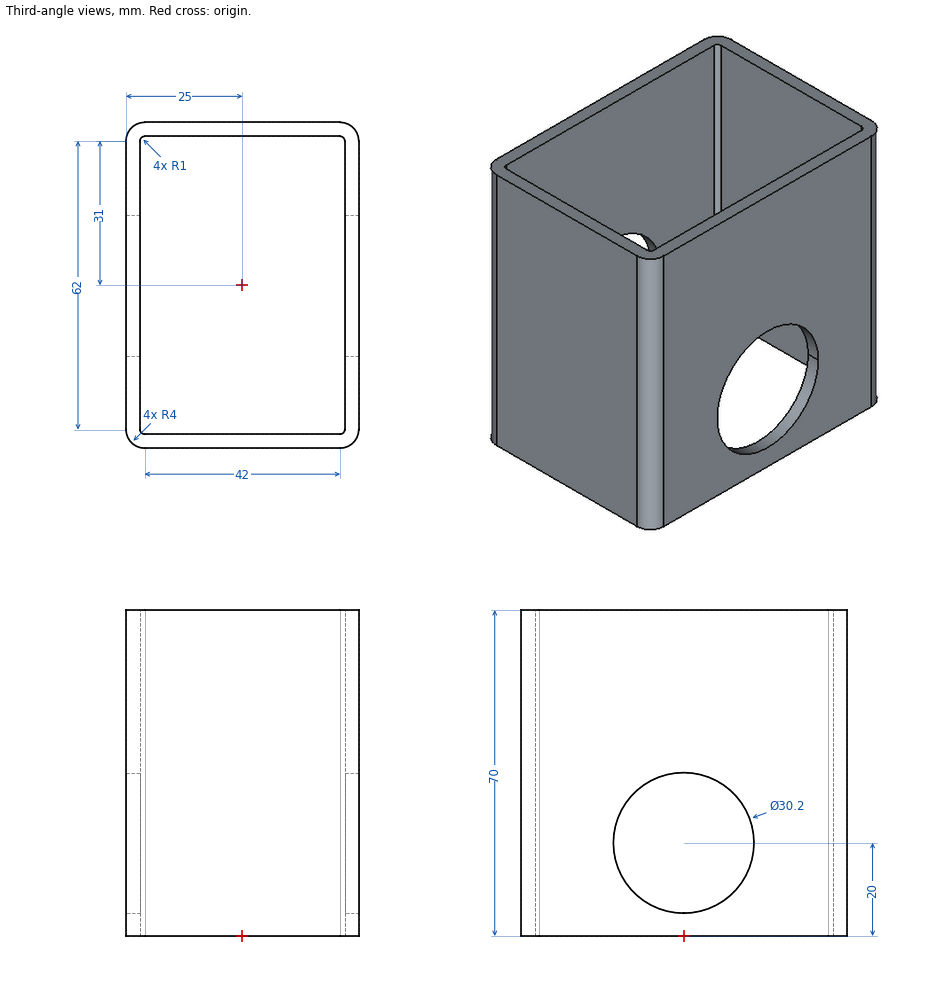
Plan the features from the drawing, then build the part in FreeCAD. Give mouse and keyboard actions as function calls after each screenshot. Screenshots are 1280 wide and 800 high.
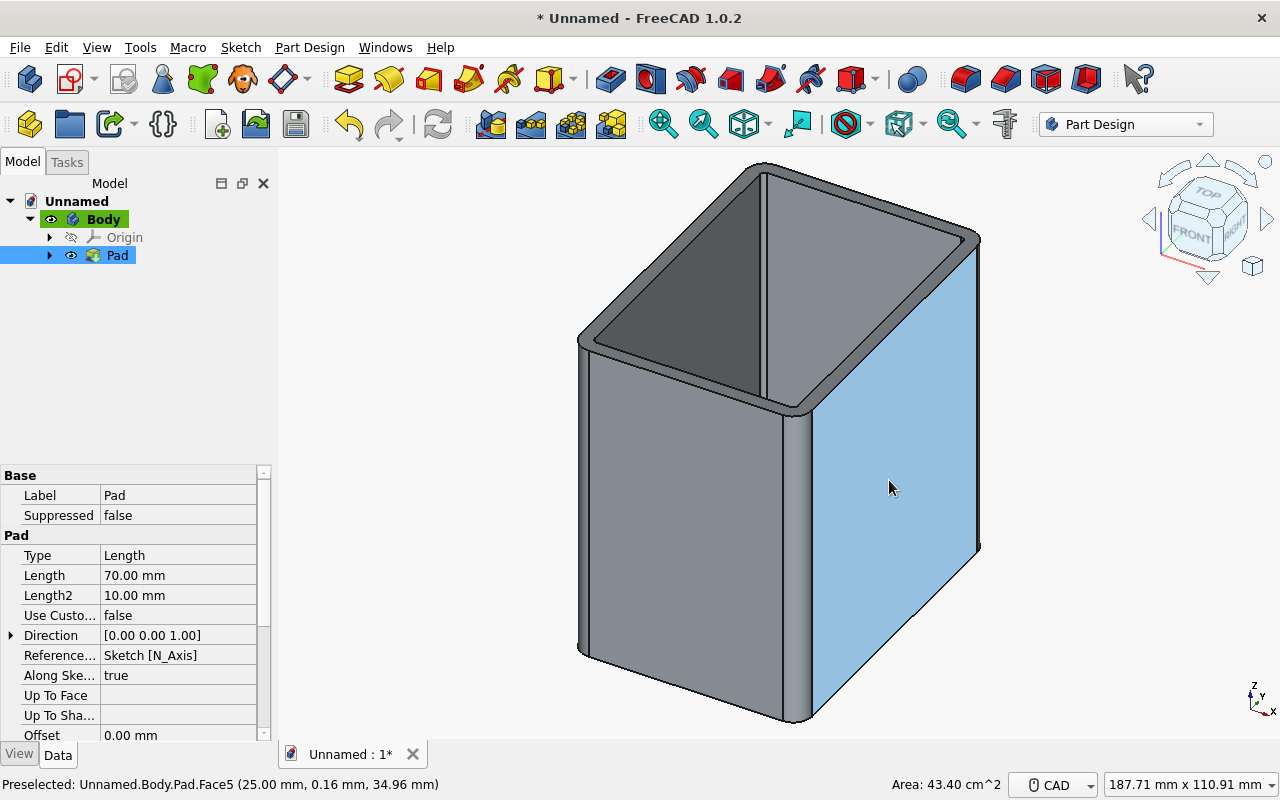
click(70, 80)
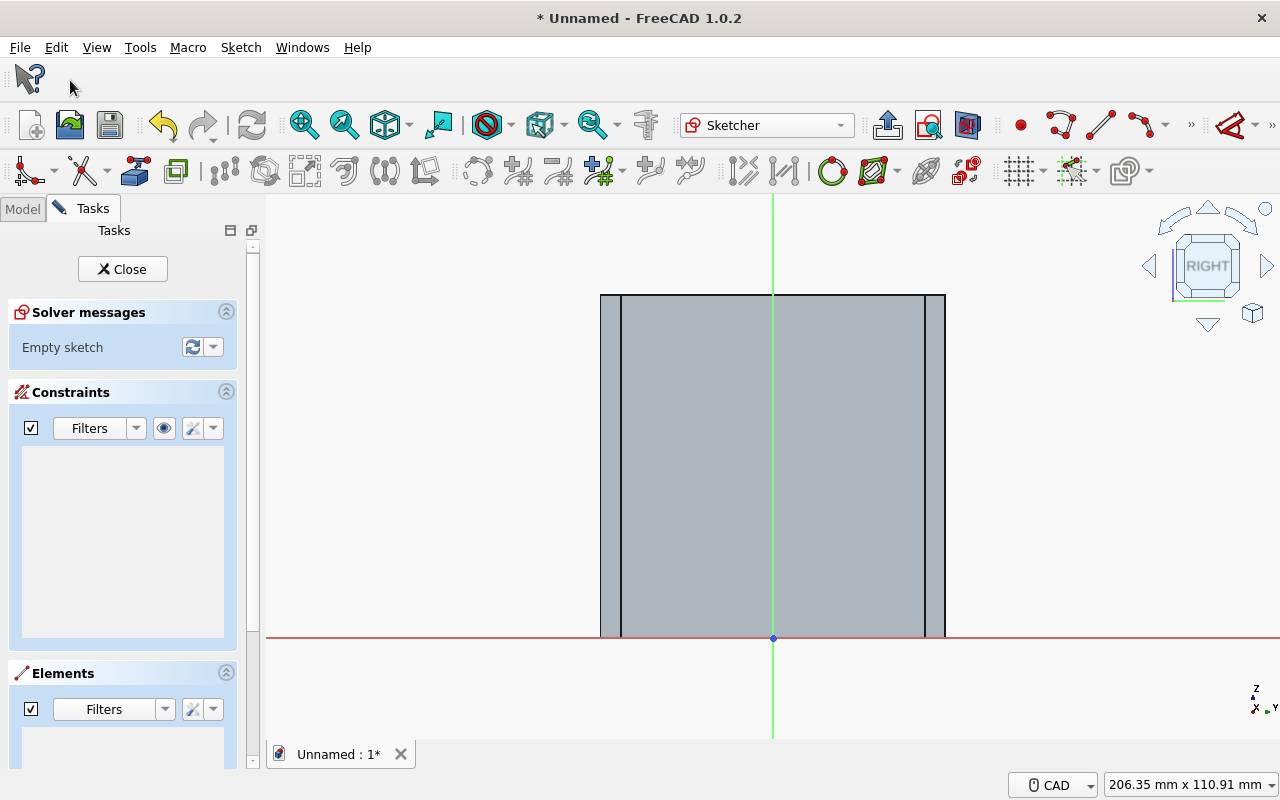
scroll(856, 657, up, 3)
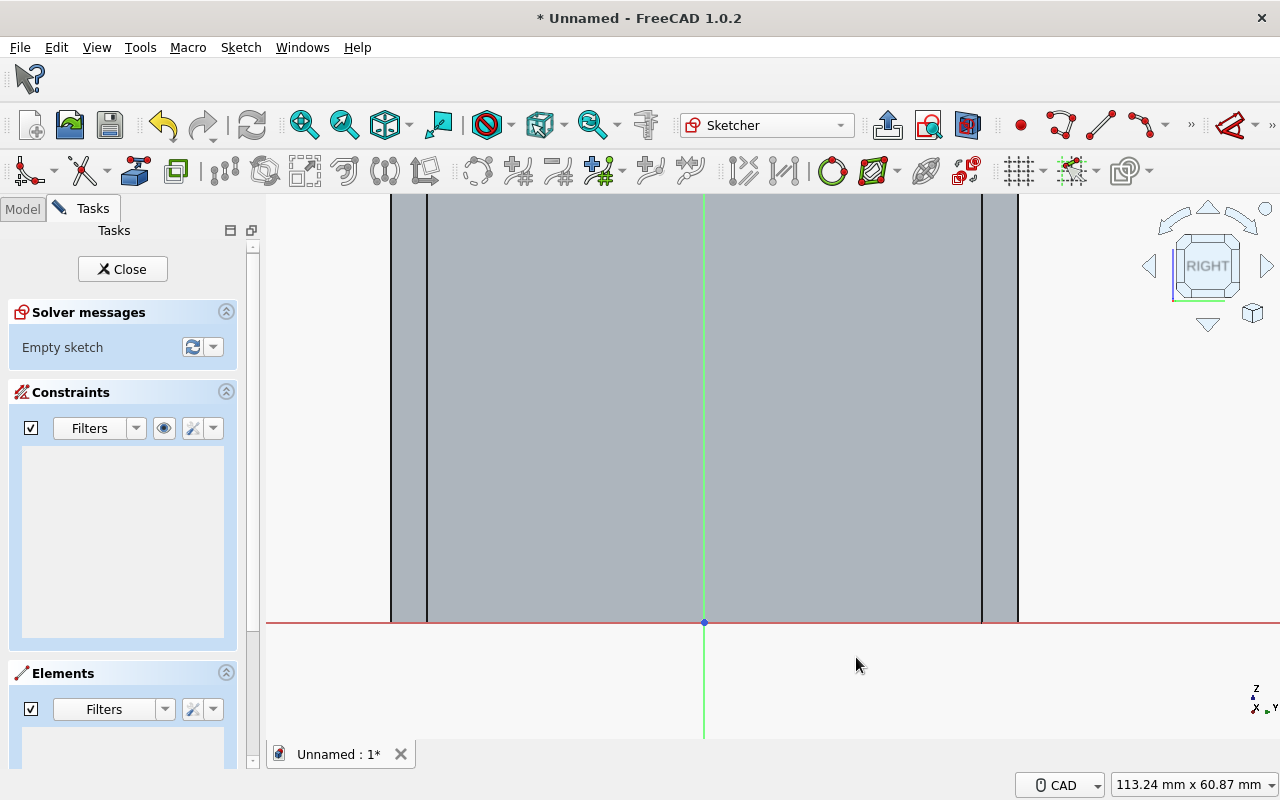
key(g)
key(c)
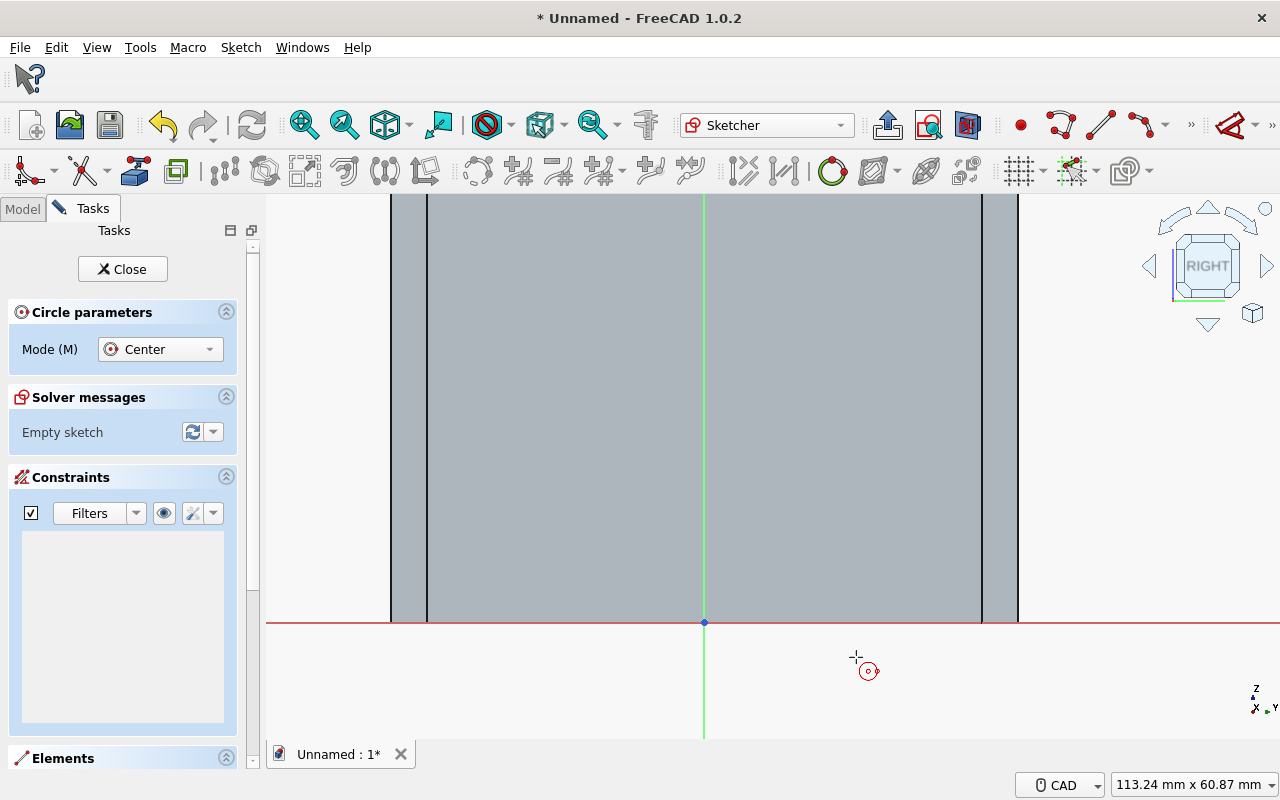
click(704, 443)
click(800, 348)
key(Escape)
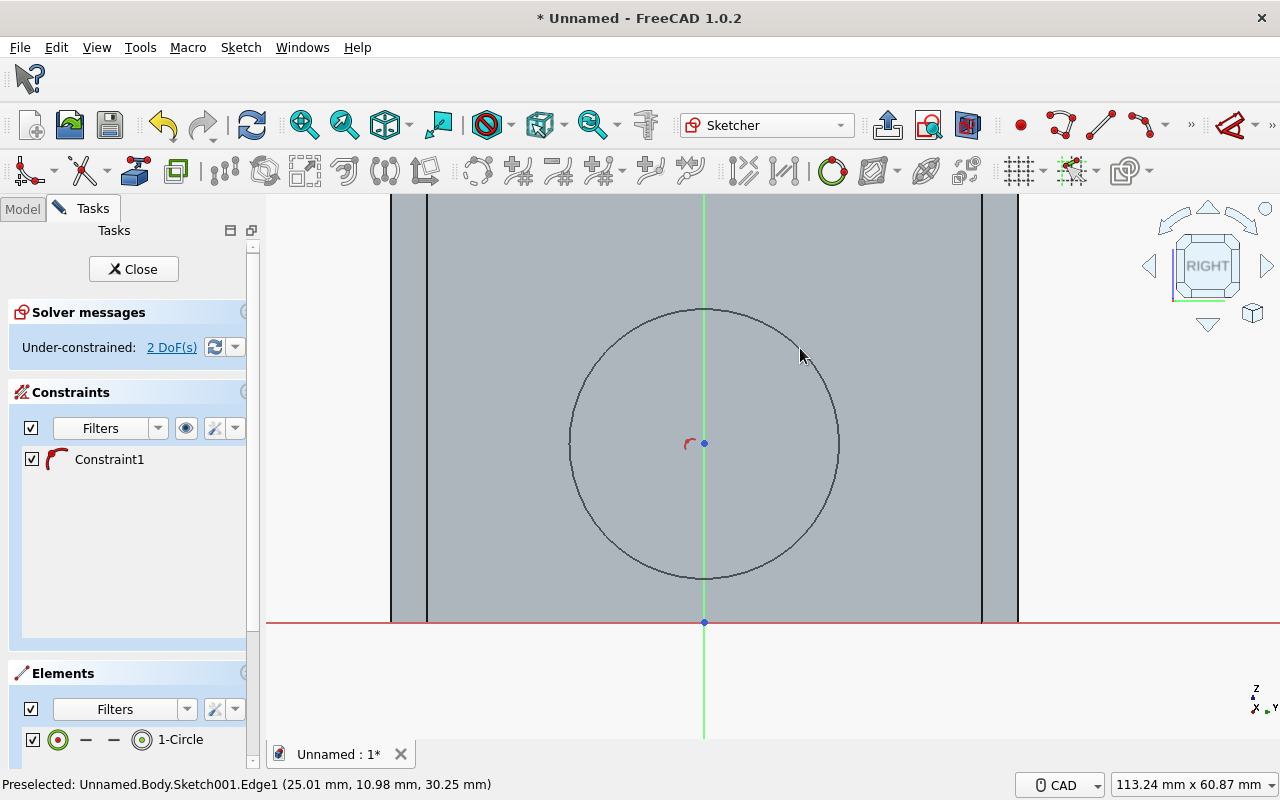
click(1230, 126)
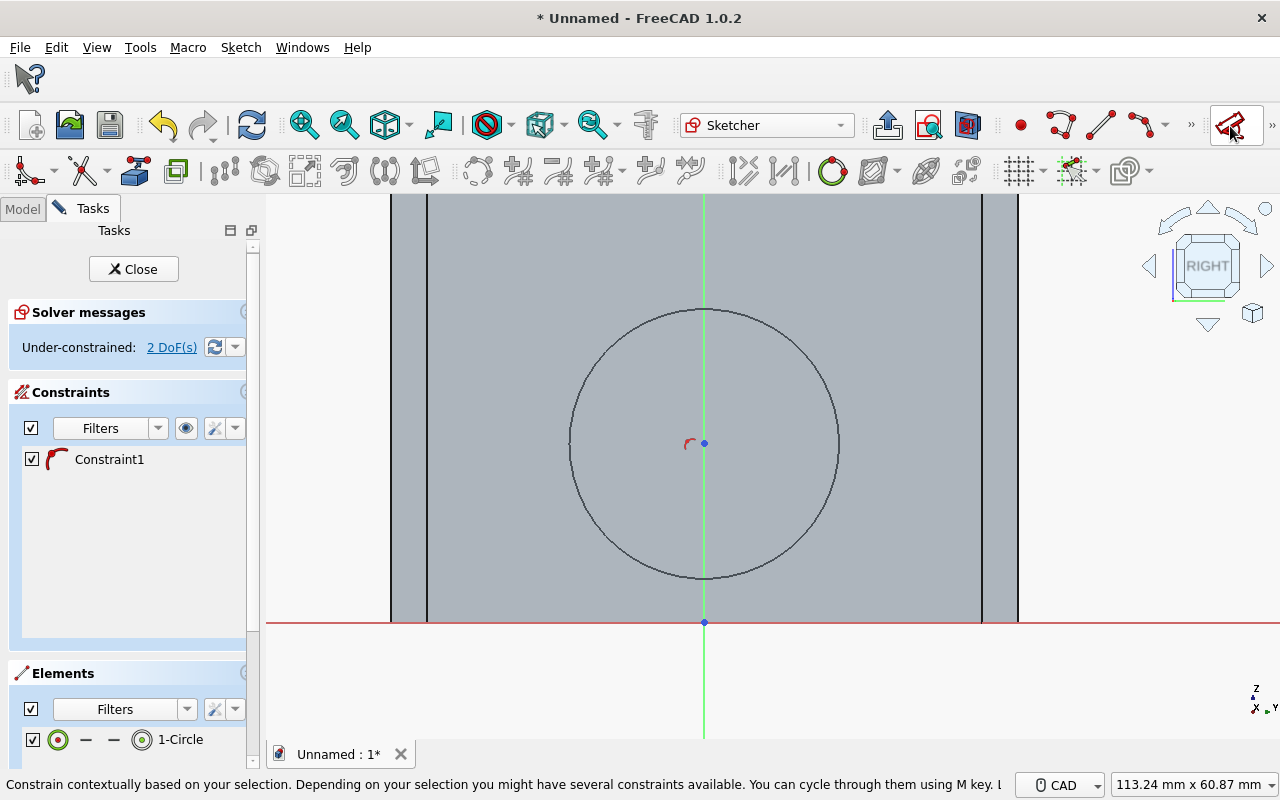
click(799, 348)
click(821, 325)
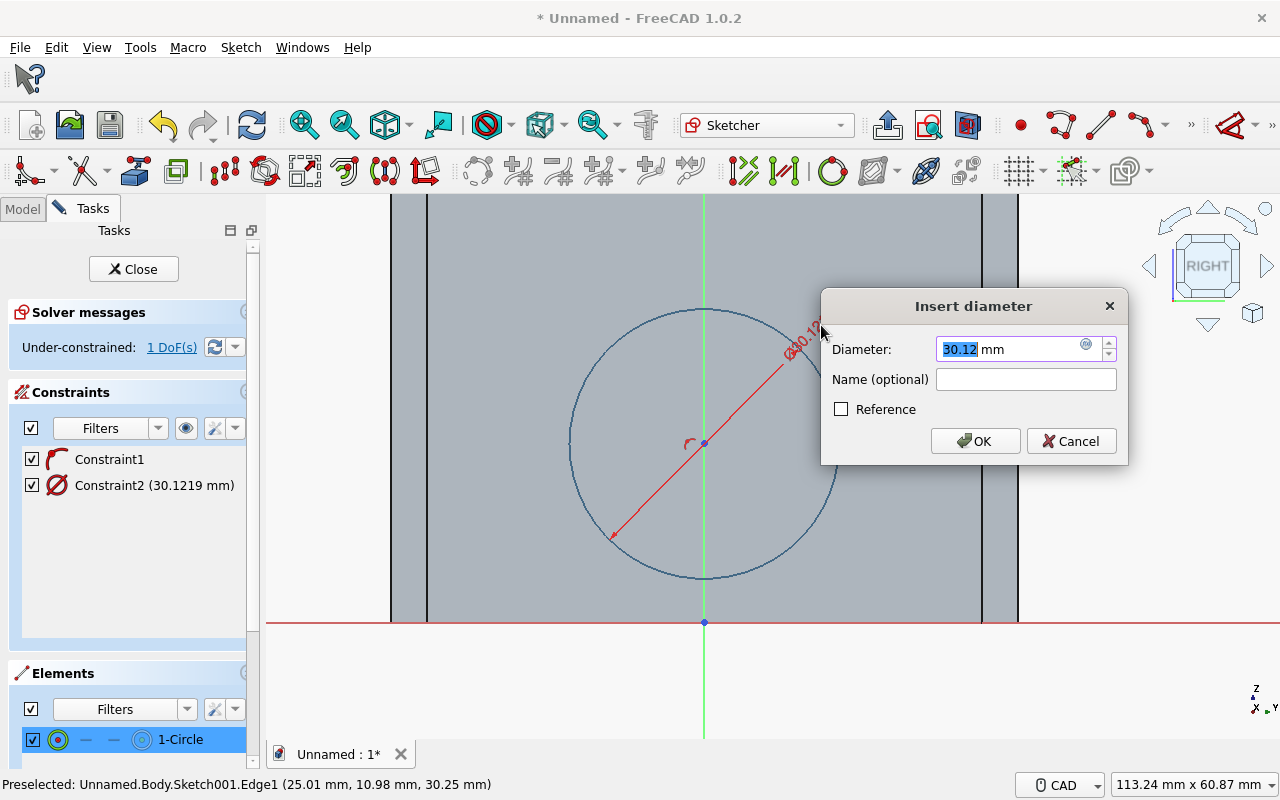
text(30.2)
key(Return)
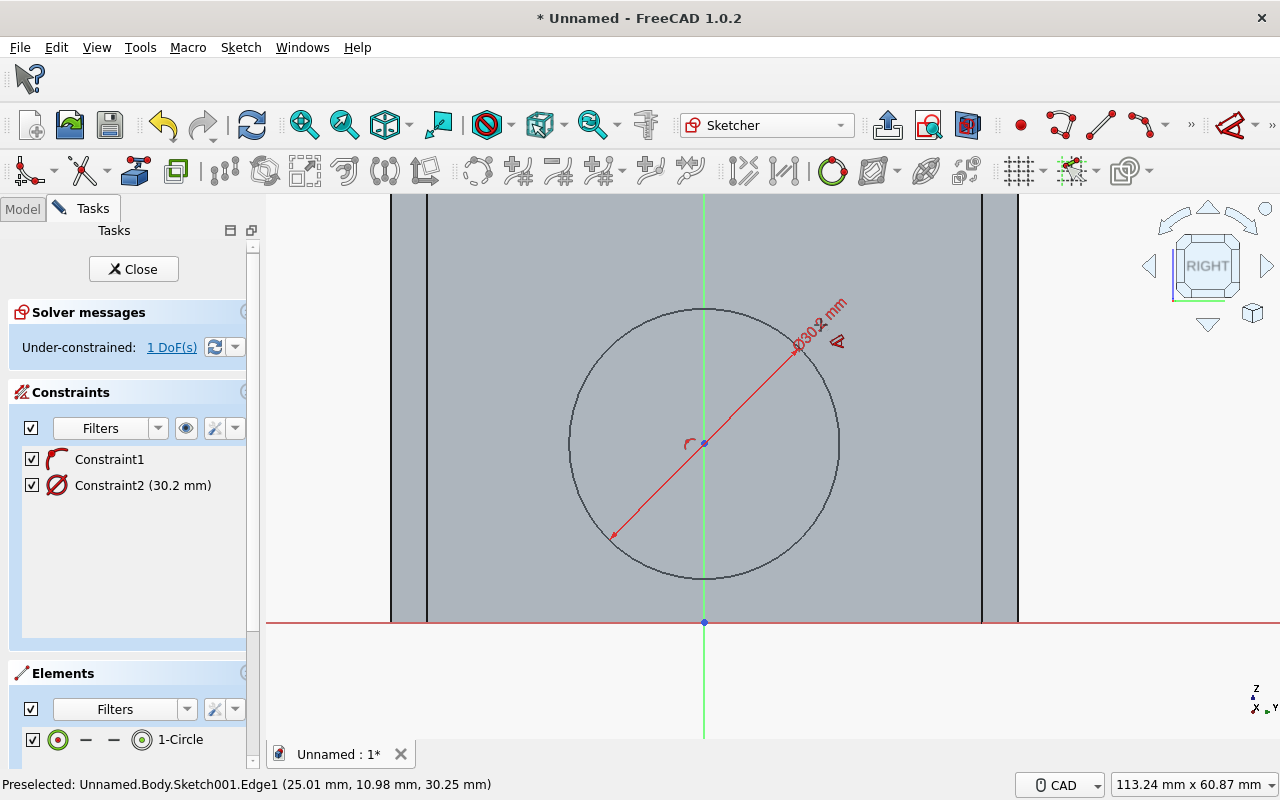
click(704, 444)
click(738, 533)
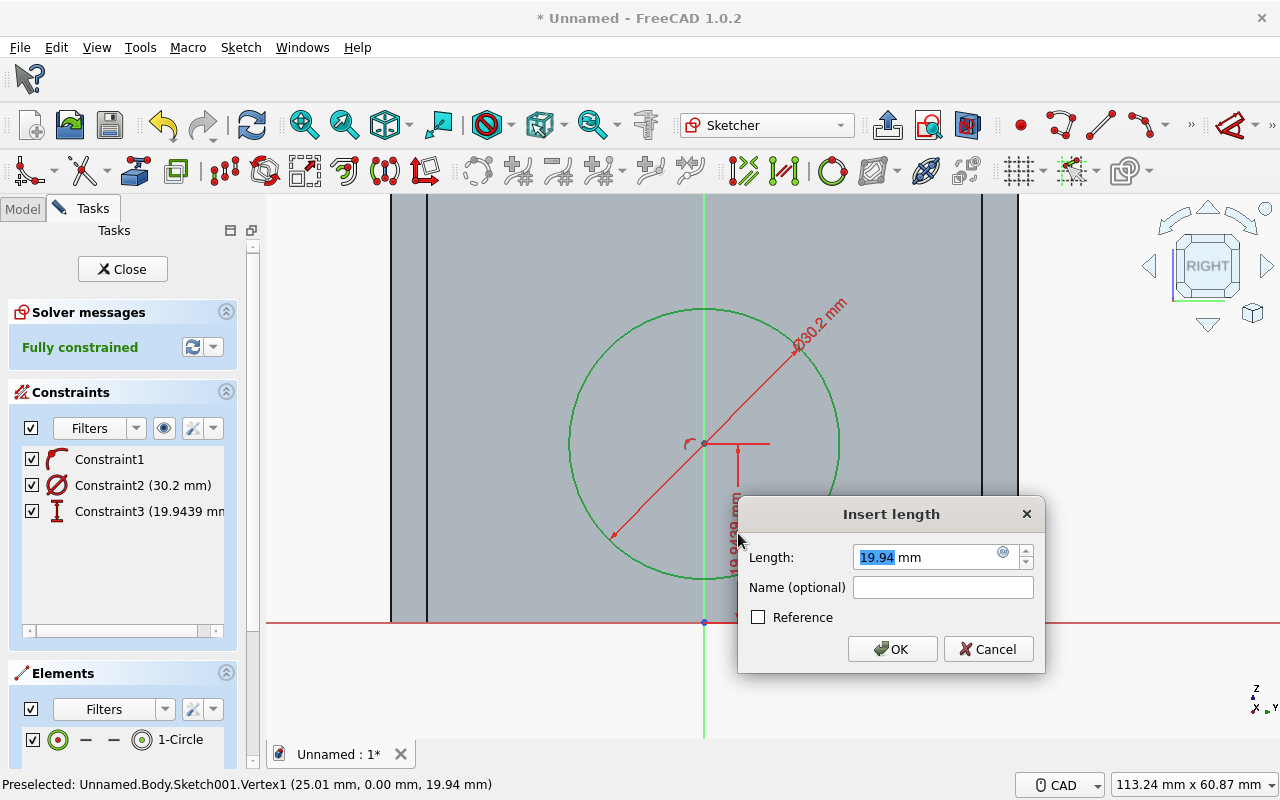
text(20)
key(Return)
key(Escape)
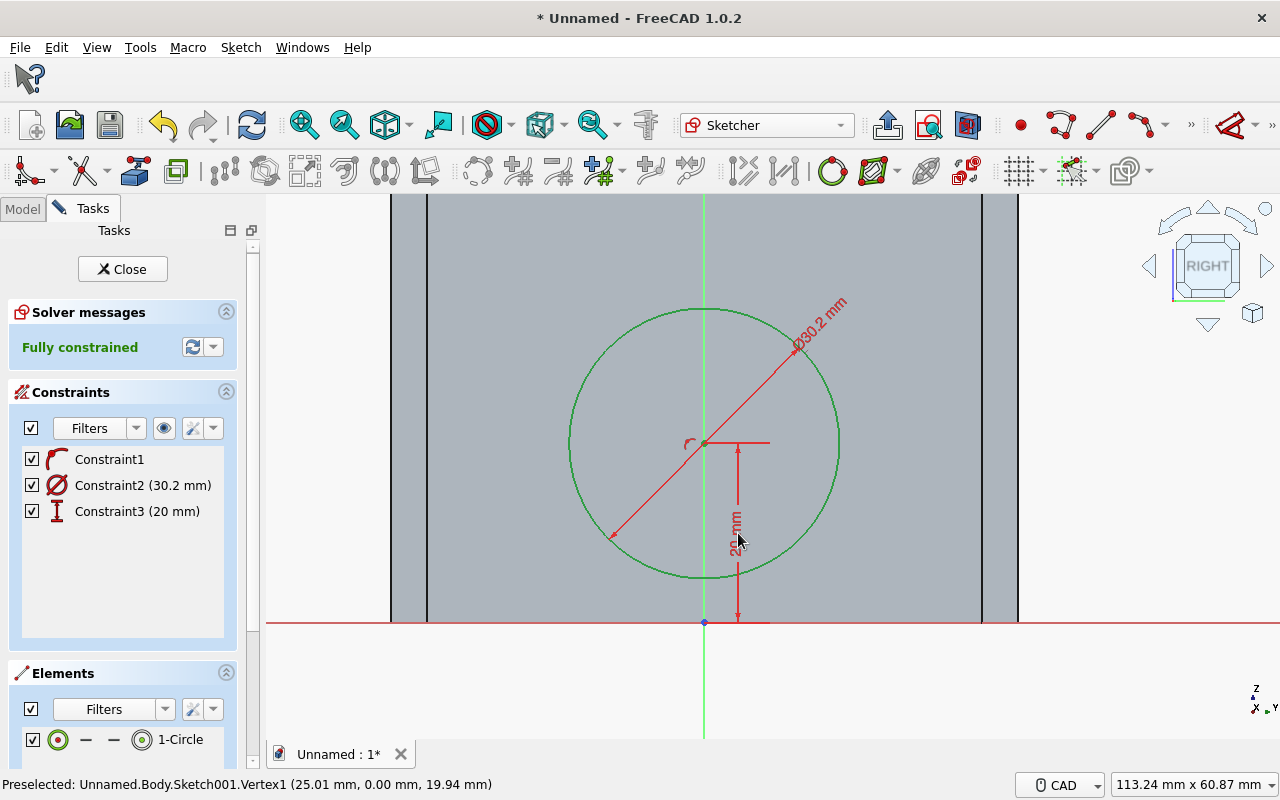
click(123, 269)